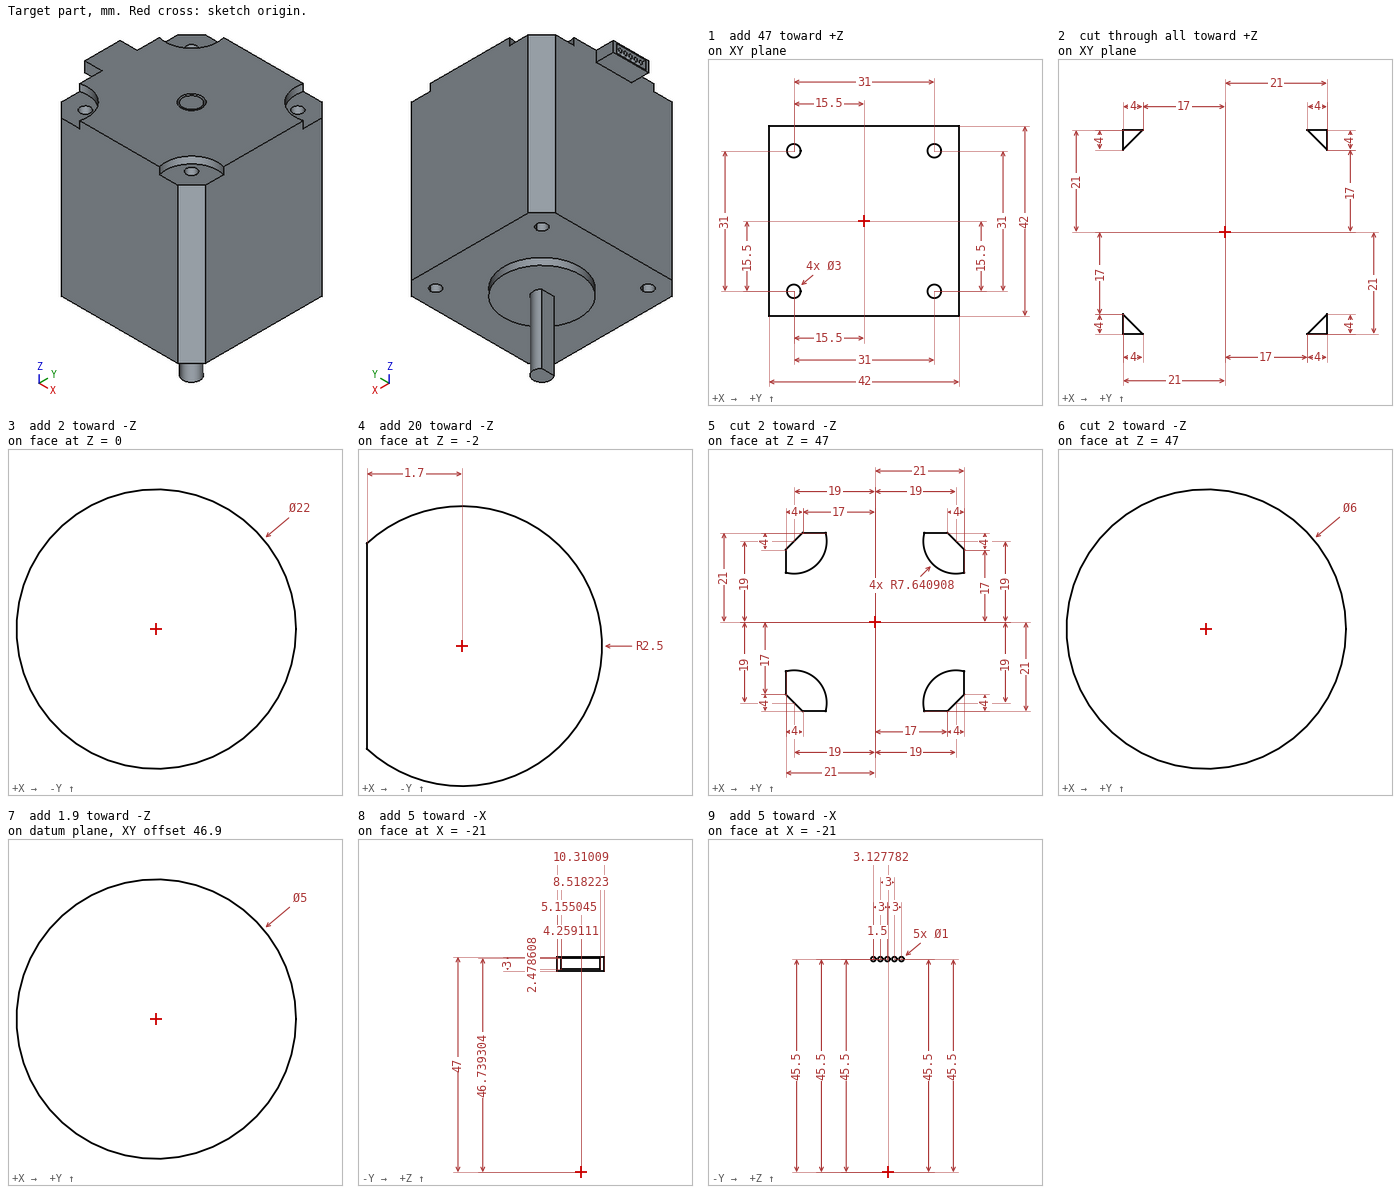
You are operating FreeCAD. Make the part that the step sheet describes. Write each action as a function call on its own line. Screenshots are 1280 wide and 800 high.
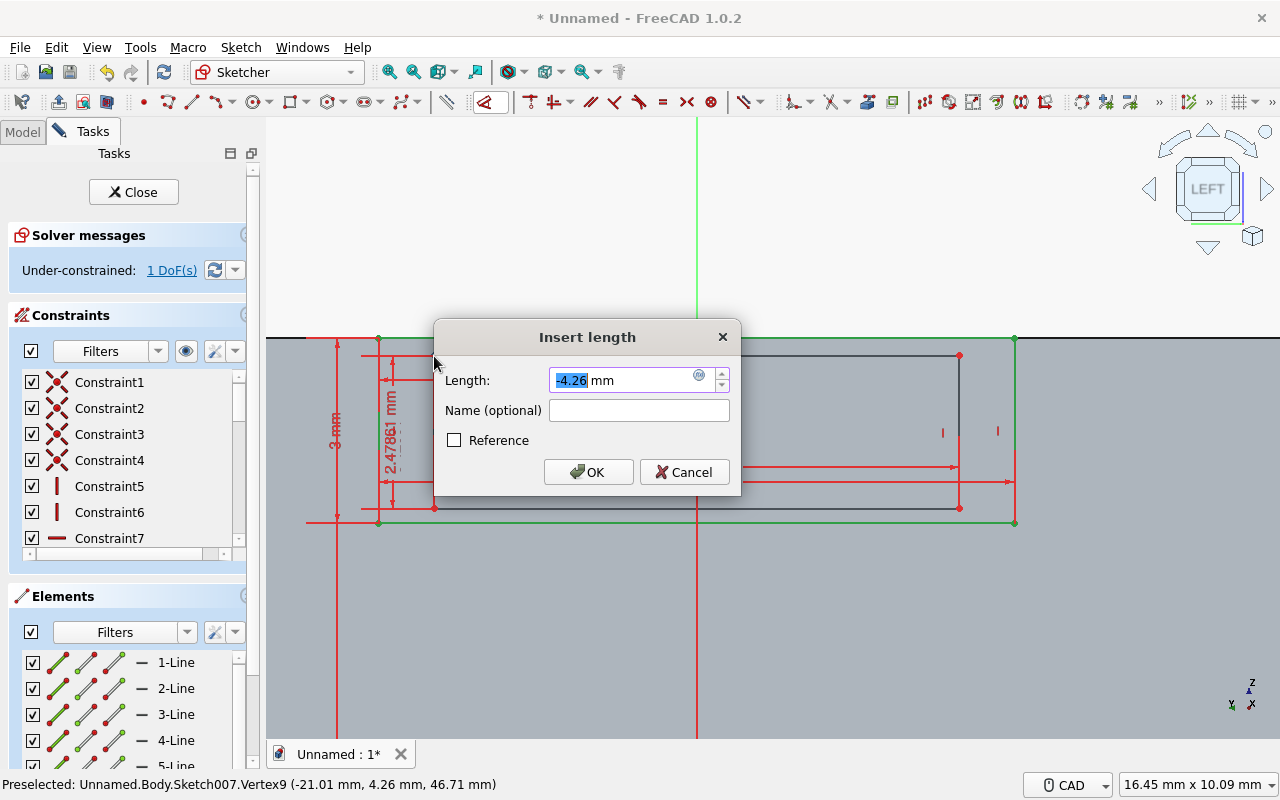
text(-4.259111)
key(Return)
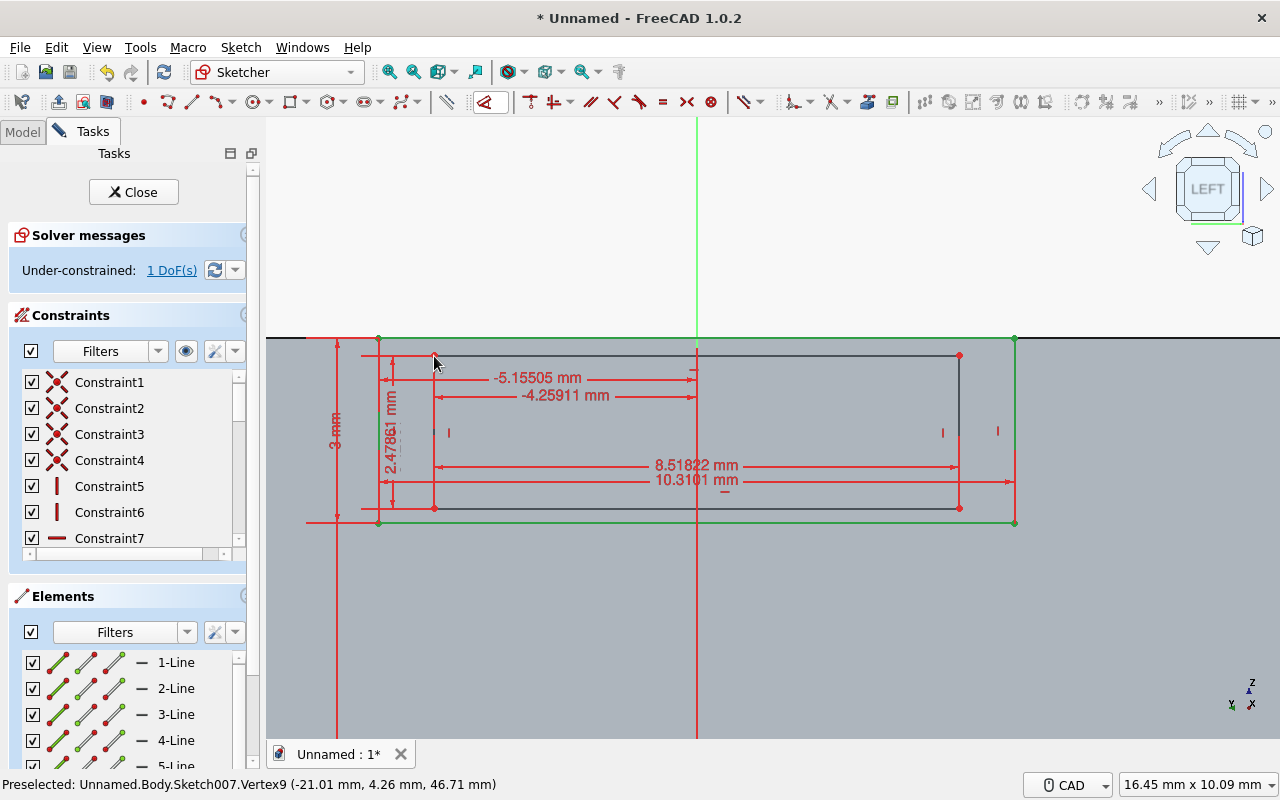
click(434, 356)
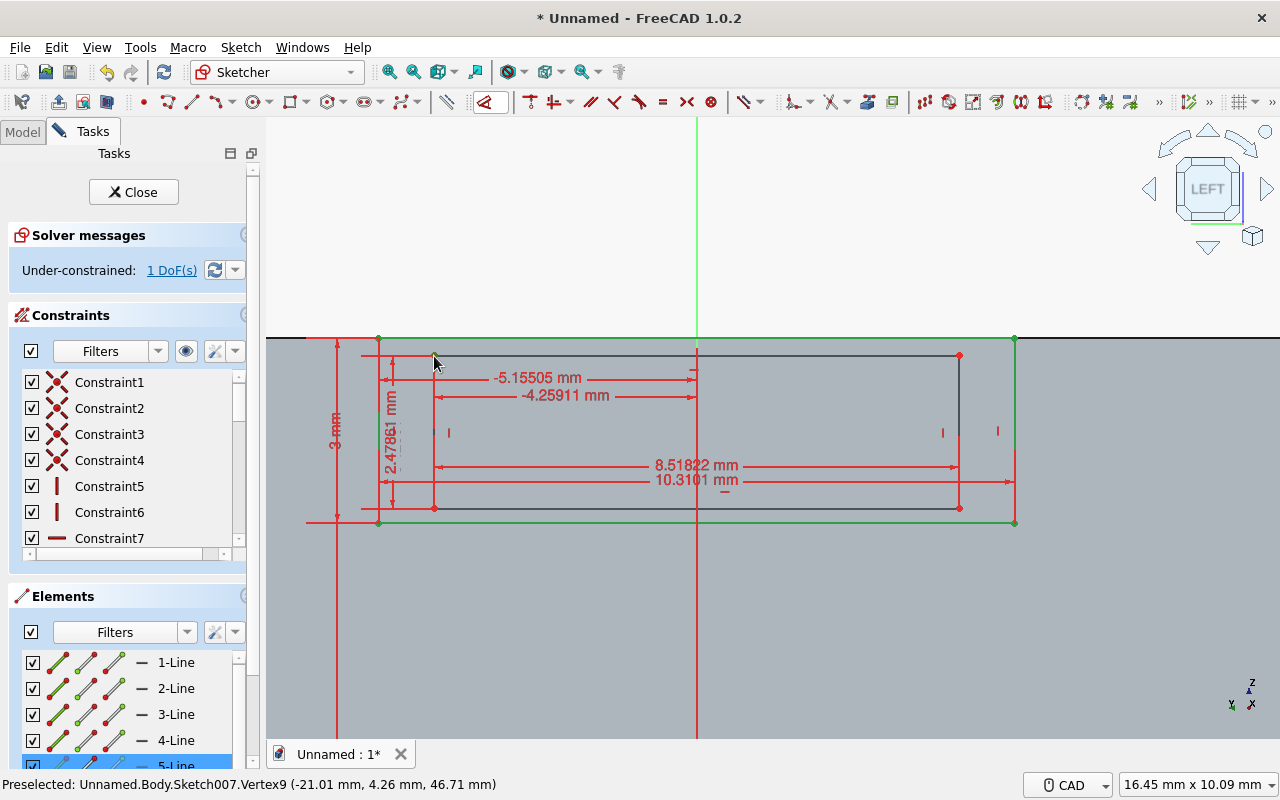
click(502, 102)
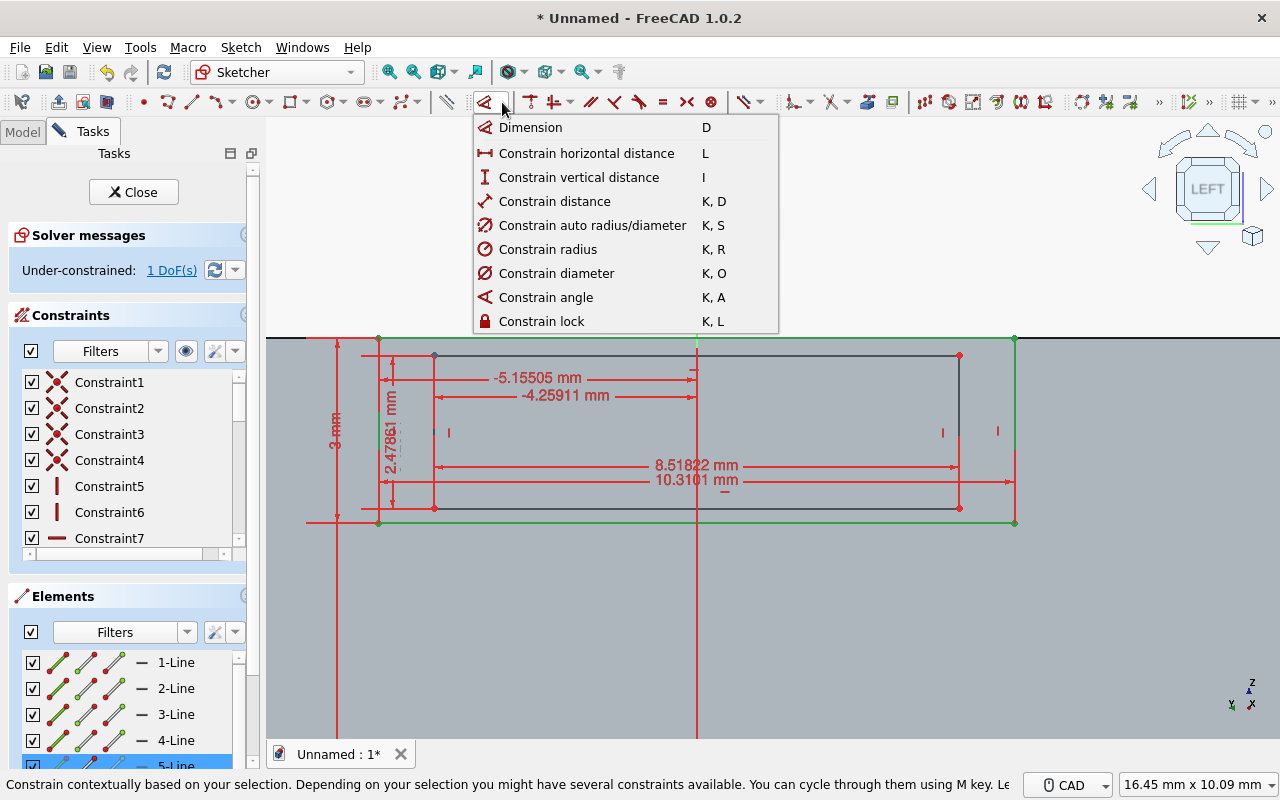
click(626, 177)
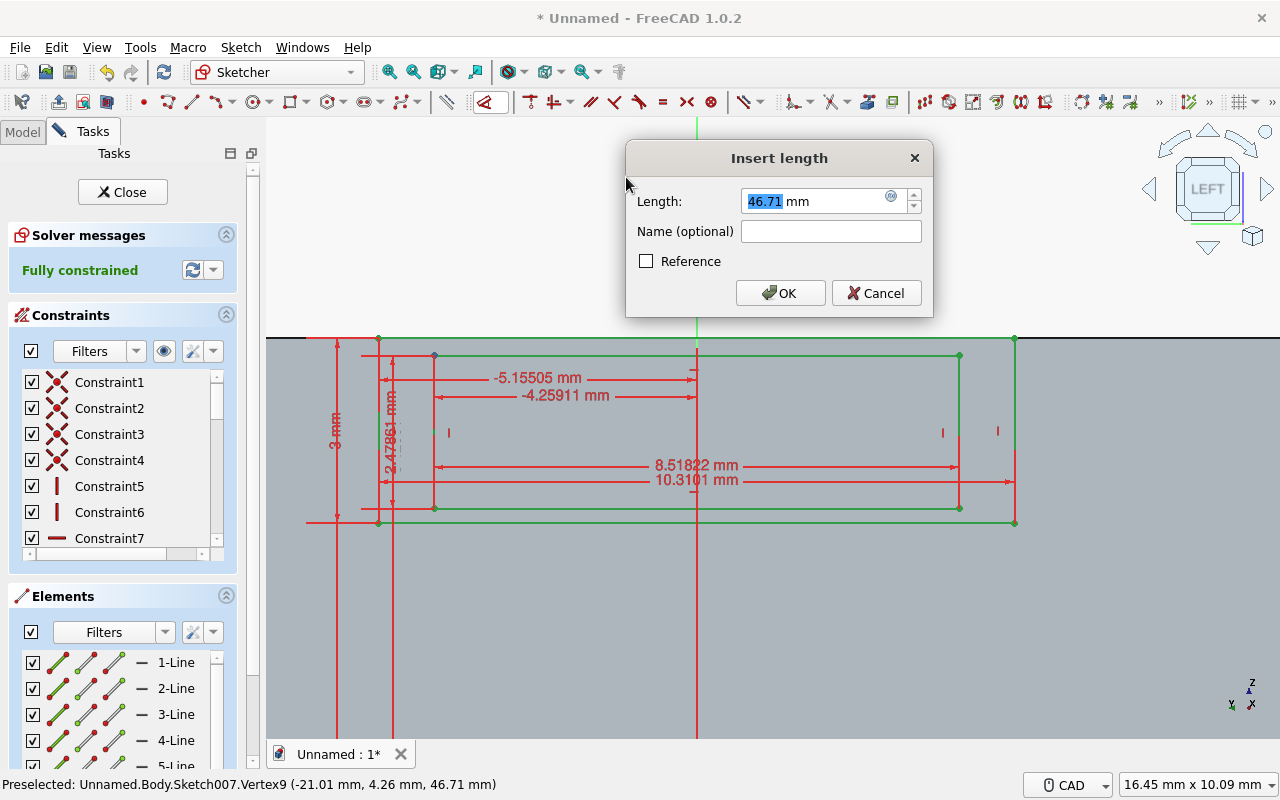
text(46.739304)
key(Return)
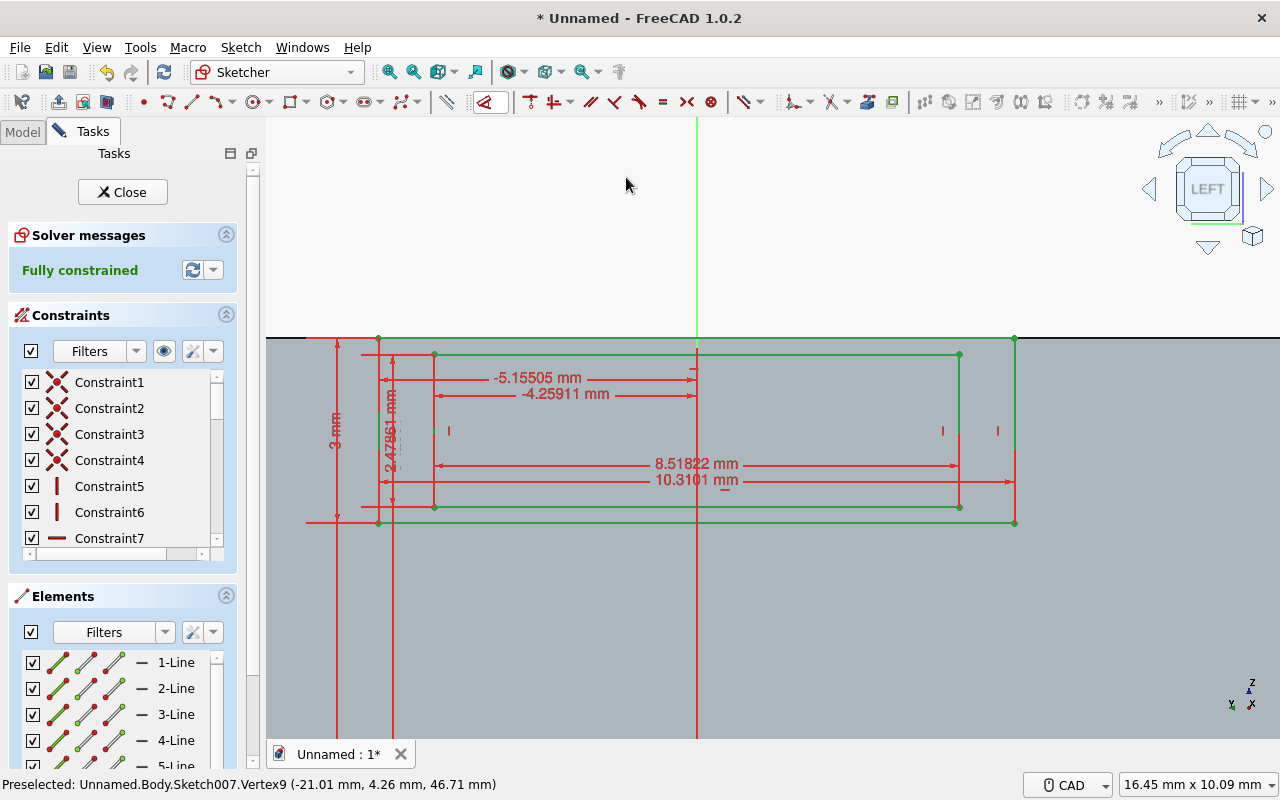
click(123, 192)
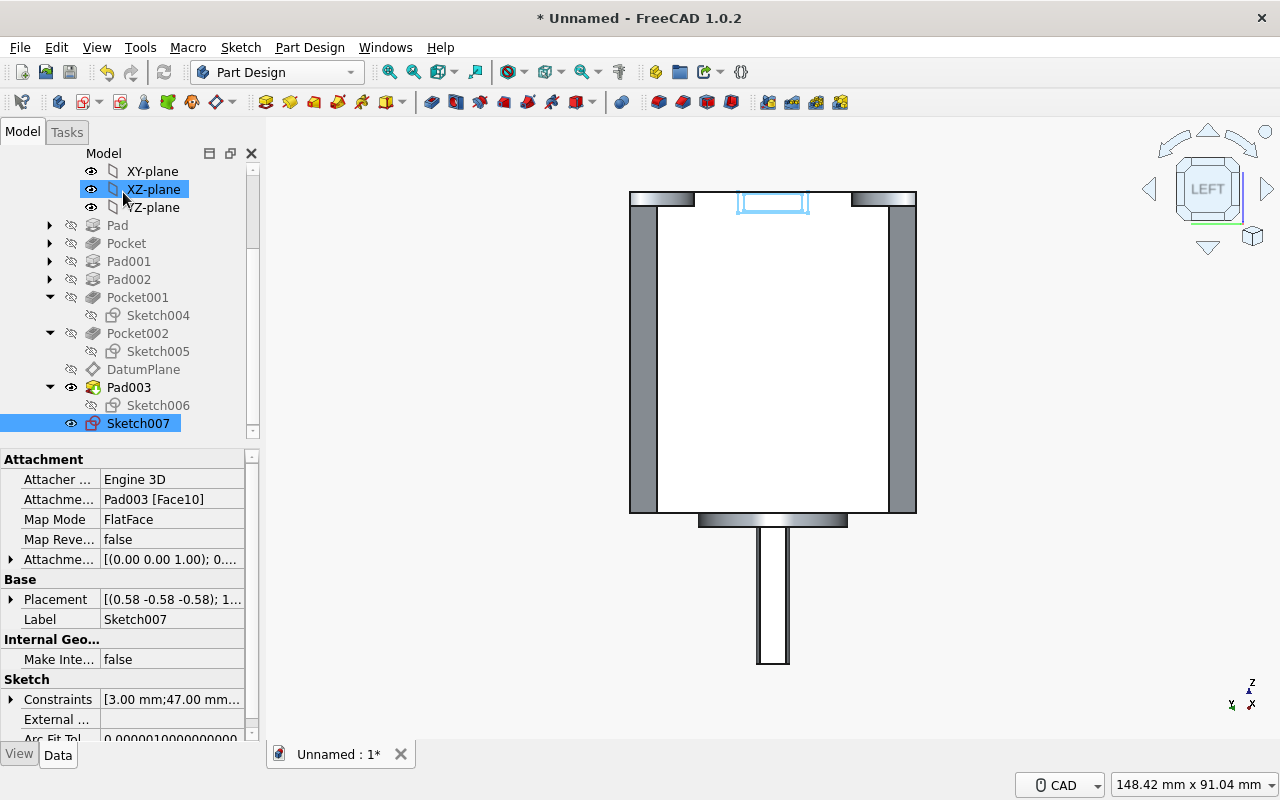
click(266, 102)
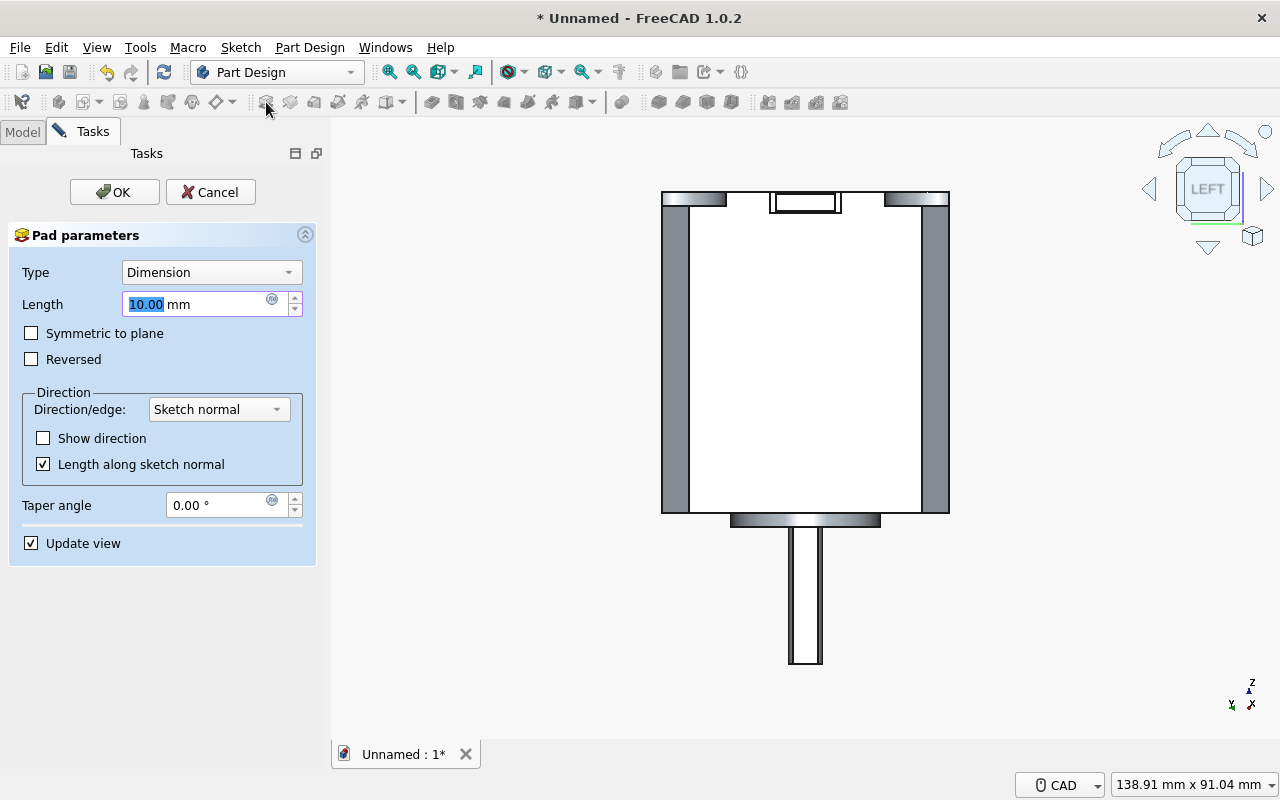
text(5)
key(Tab)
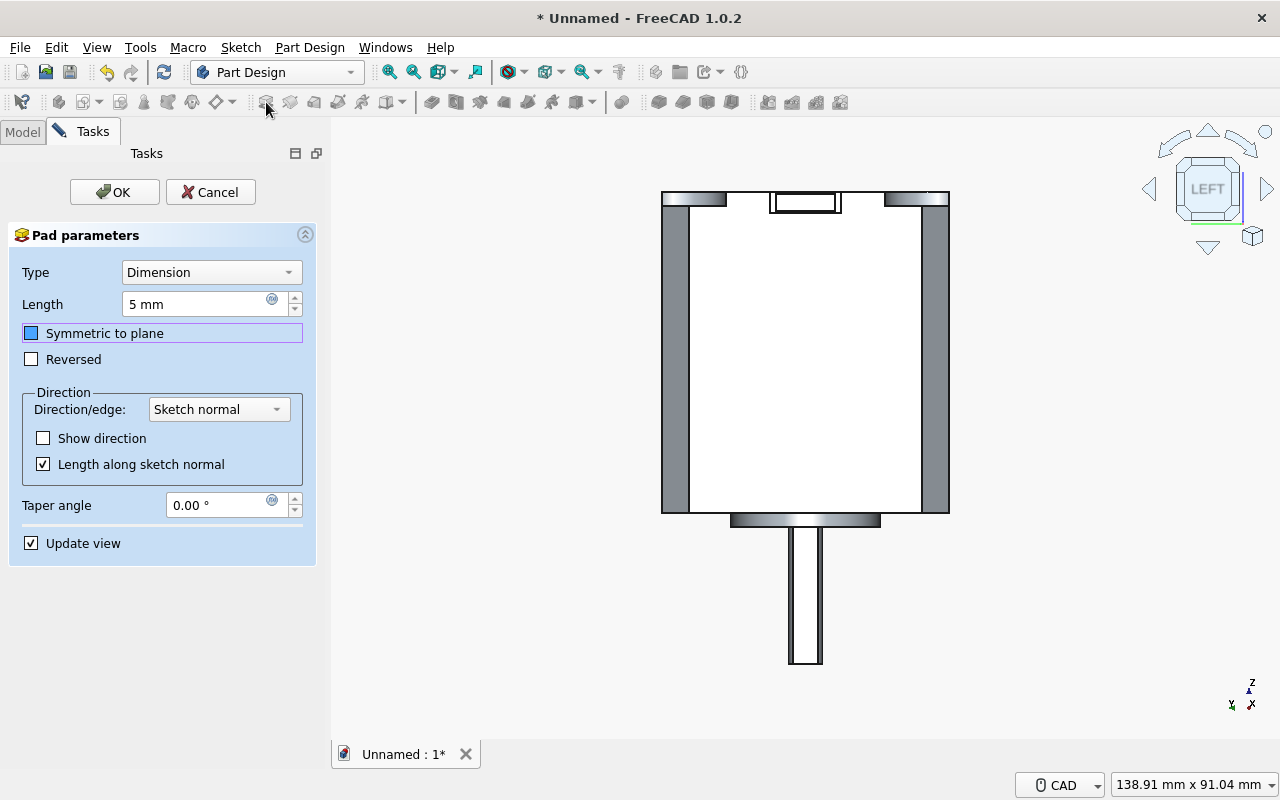
click(115, 192)